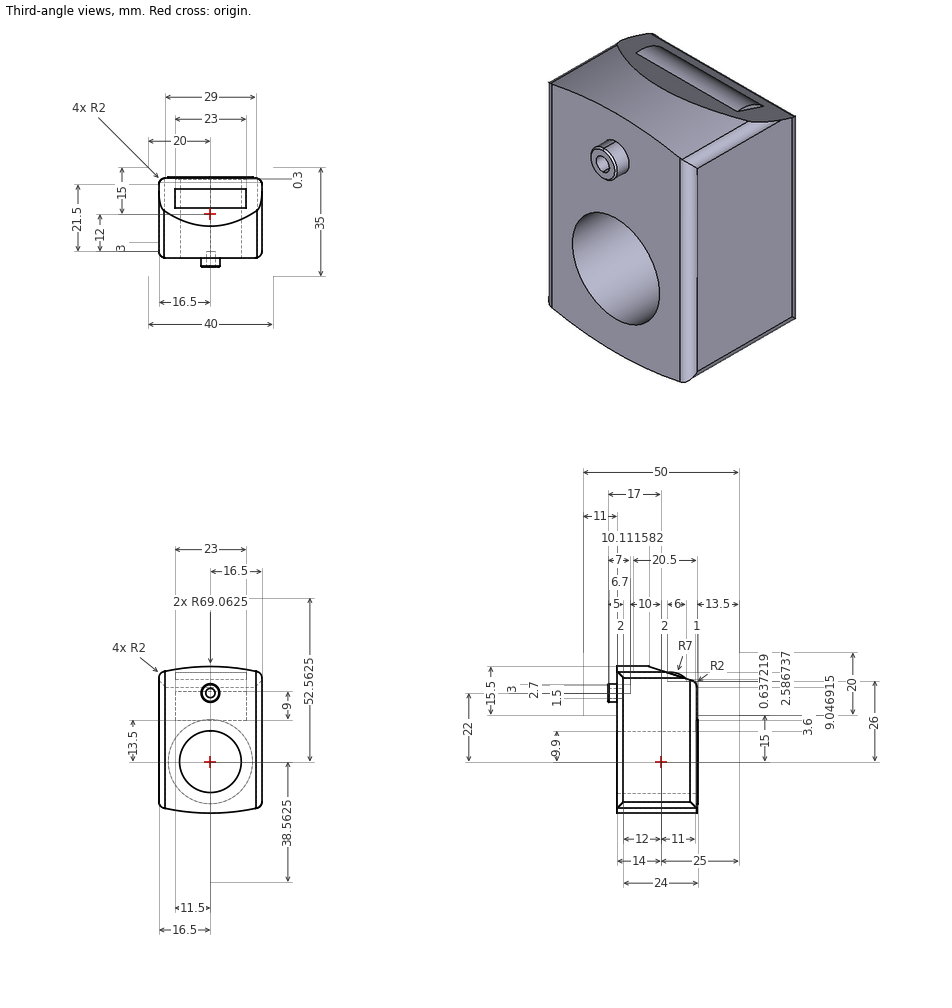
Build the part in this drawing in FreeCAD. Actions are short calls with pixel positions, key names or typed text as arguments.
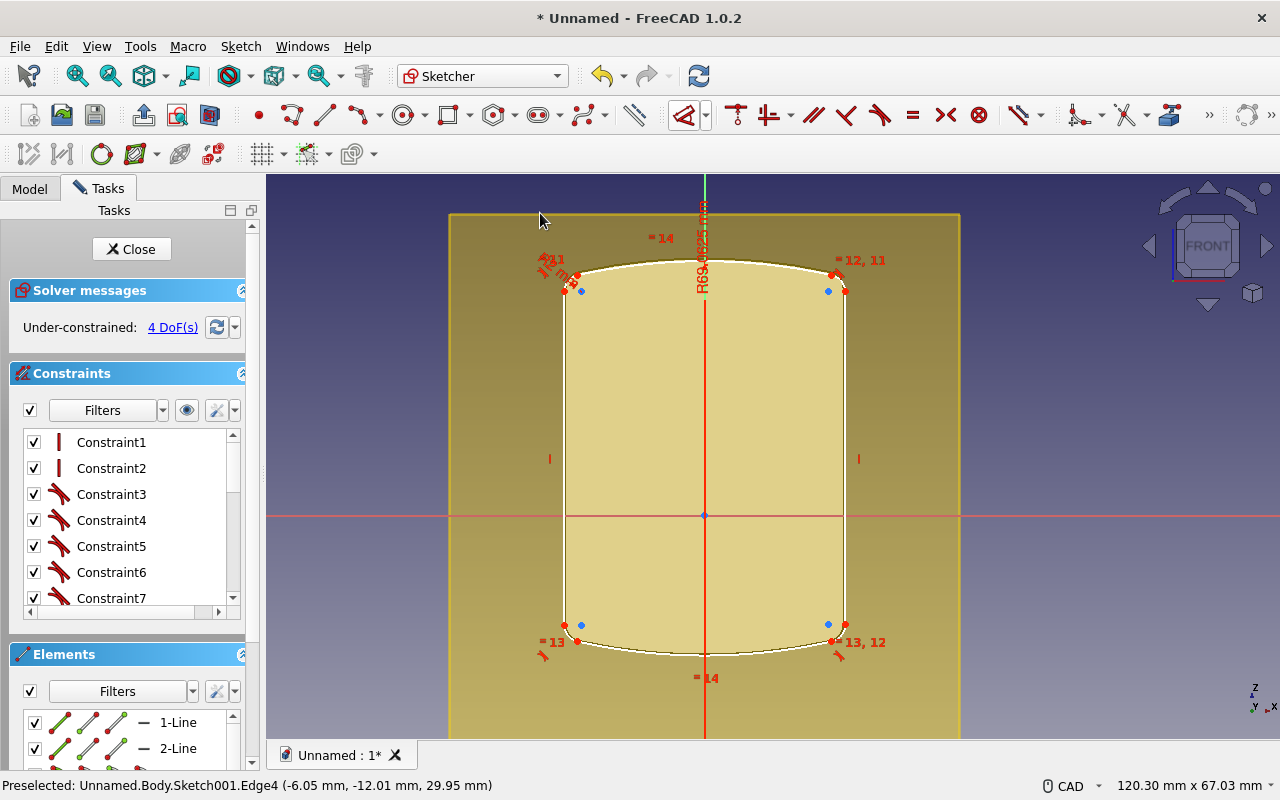
click(564, 625)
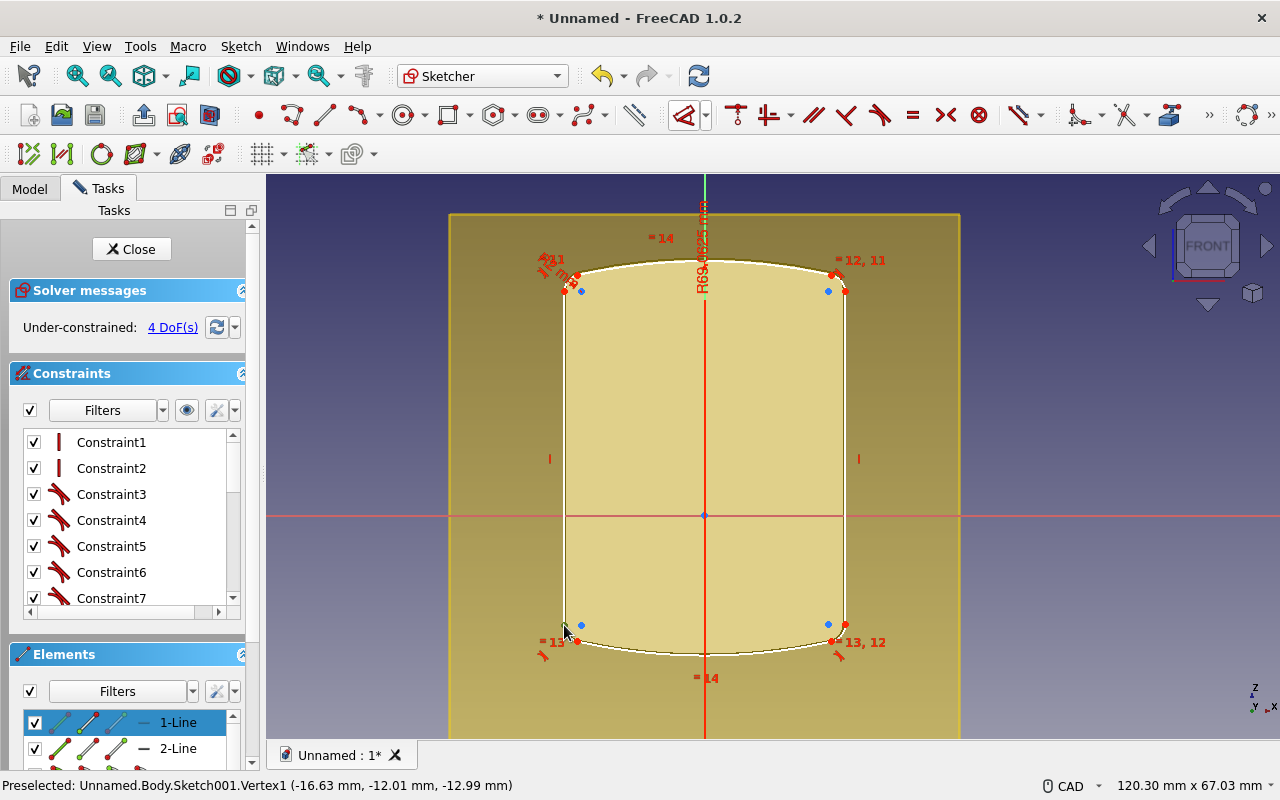
click(706, 116)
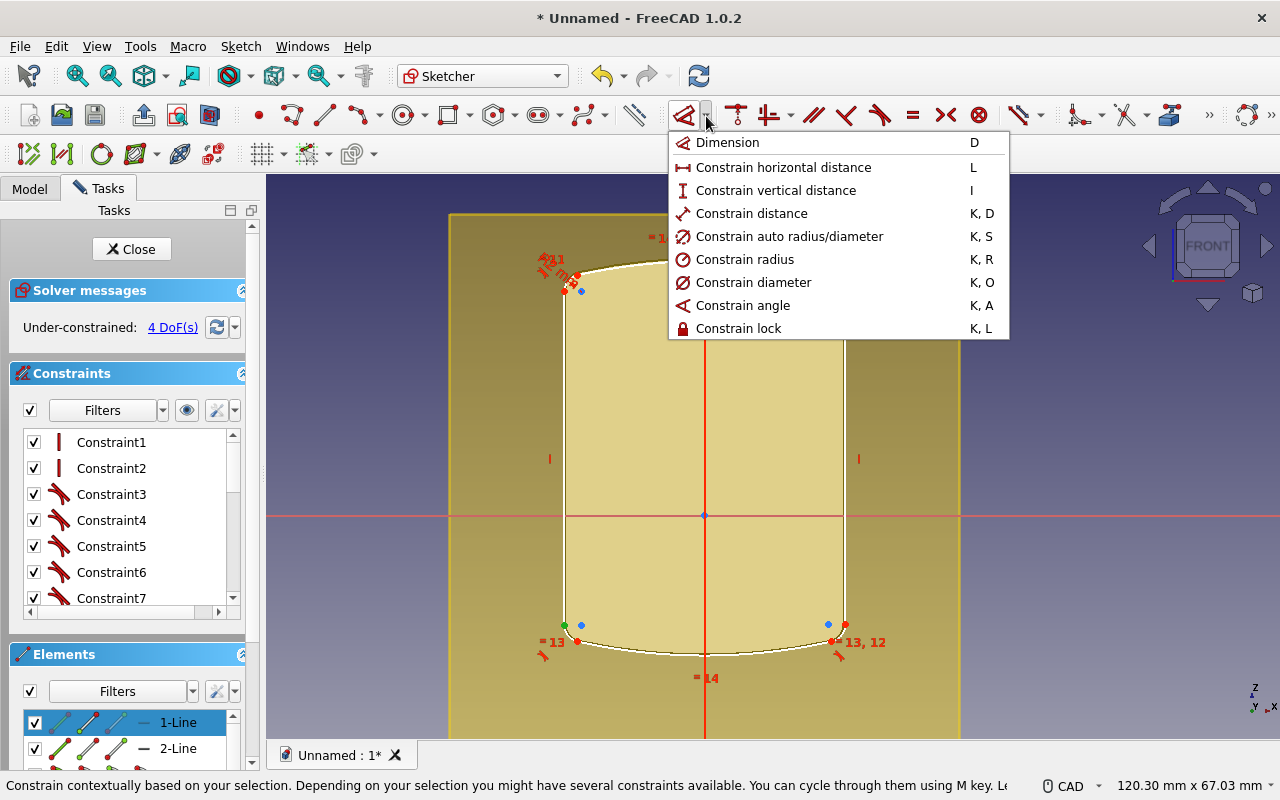
click(839, 168)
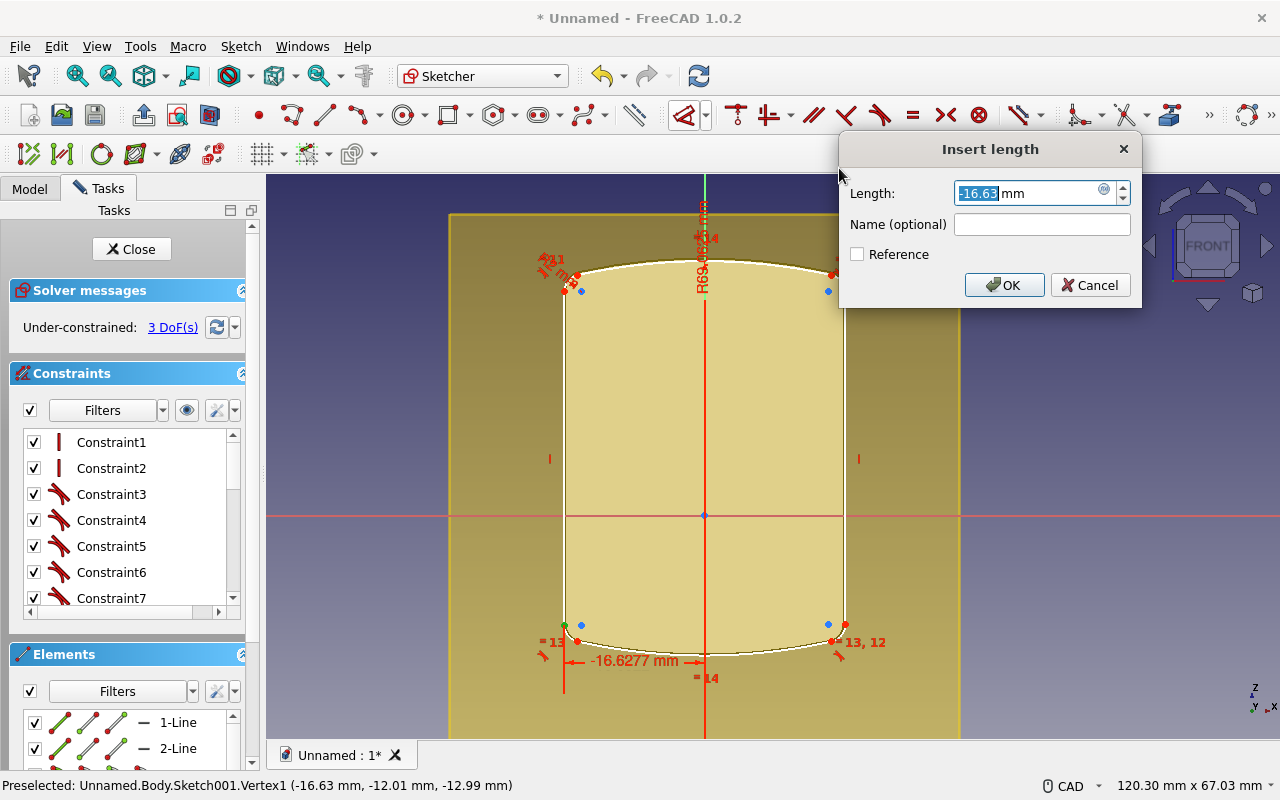
text(-16.5)
key(Return)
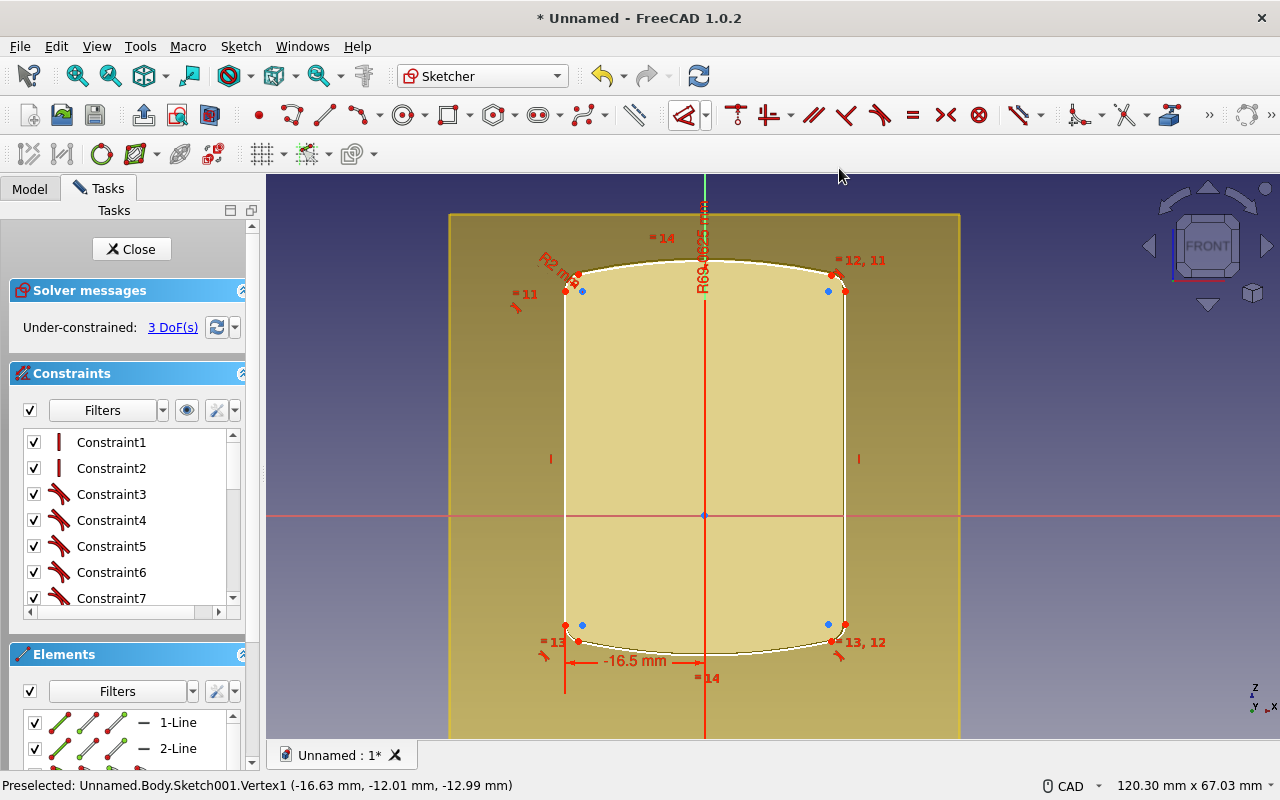
click(845, 292)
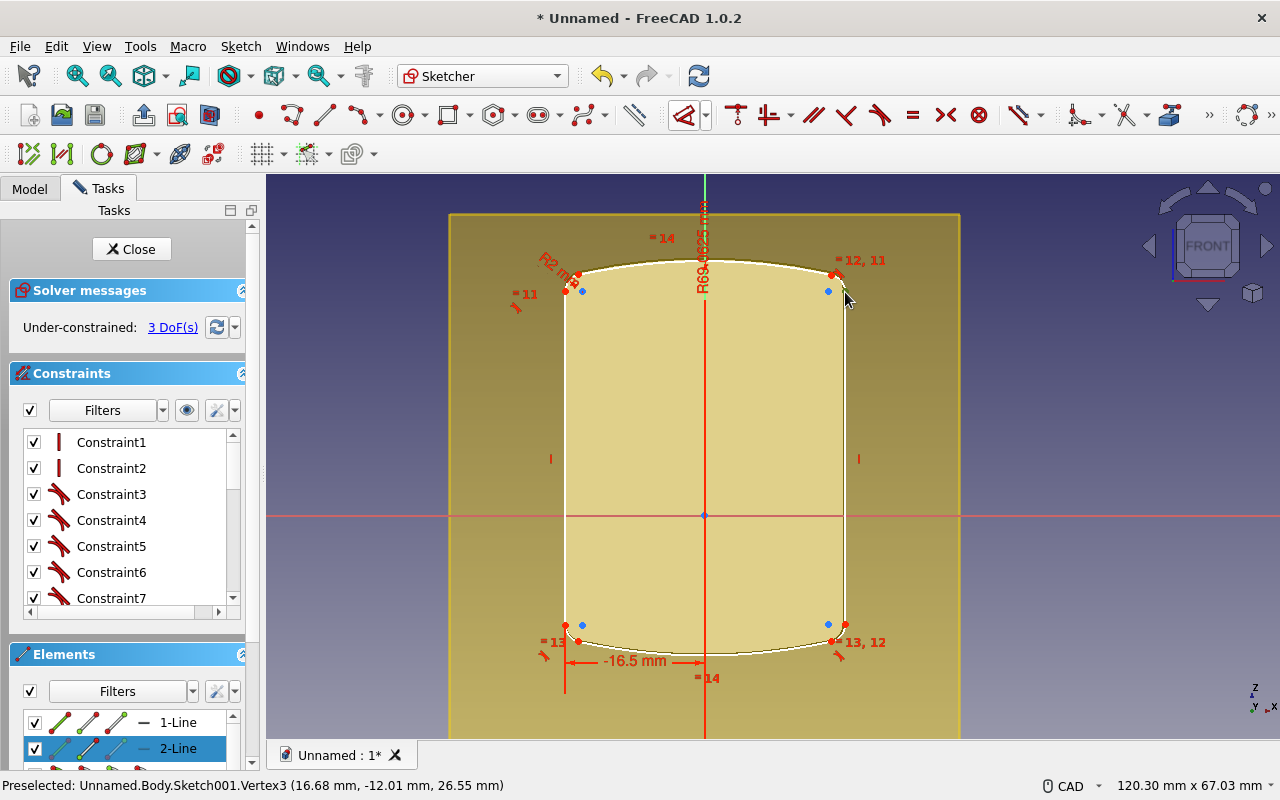
key(l)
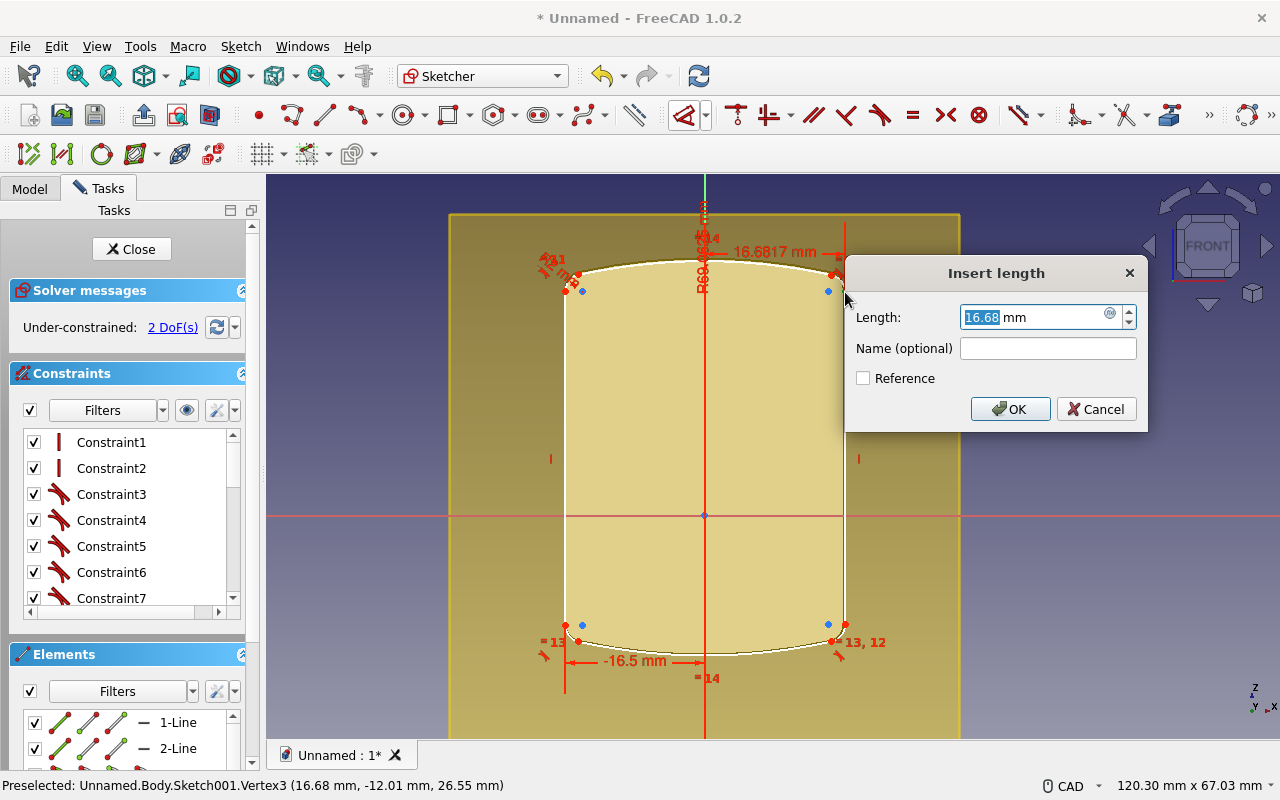
text(16.5)
key(Return)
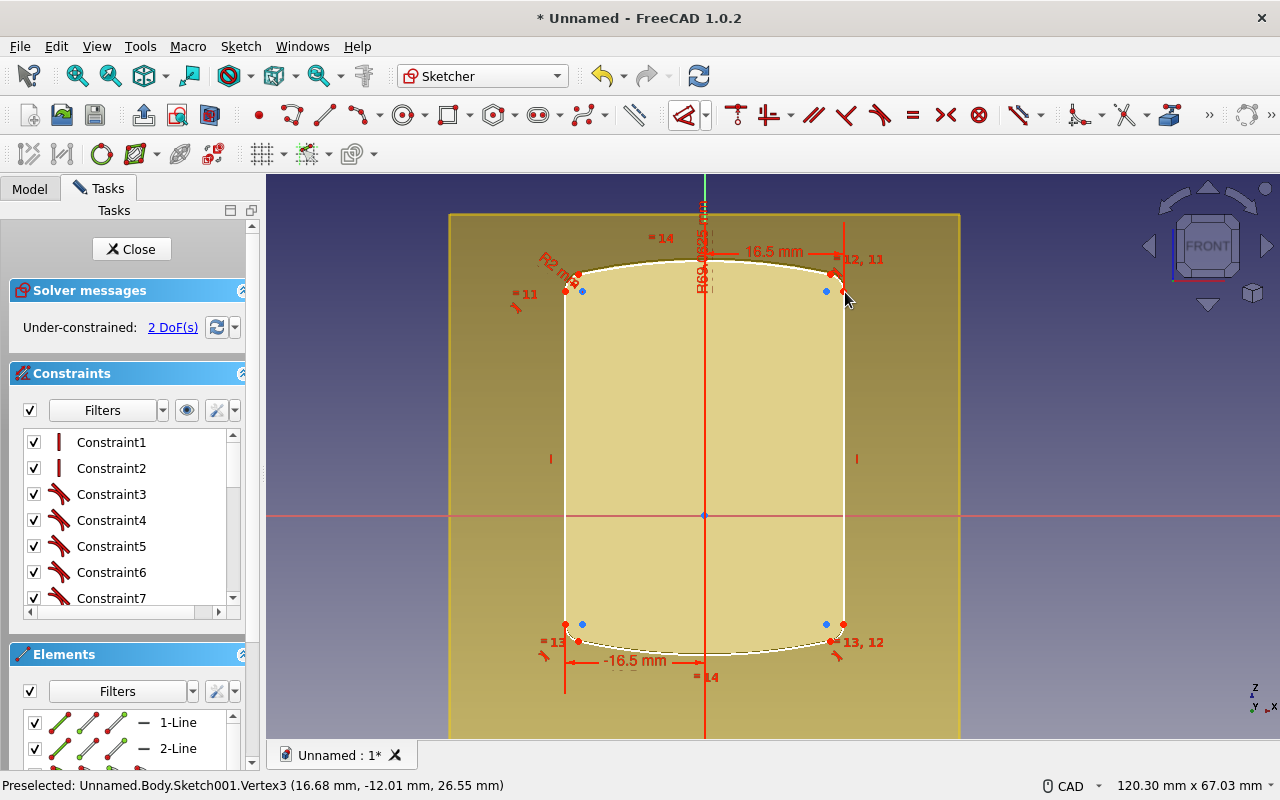
scroll(704, 265, down, 2)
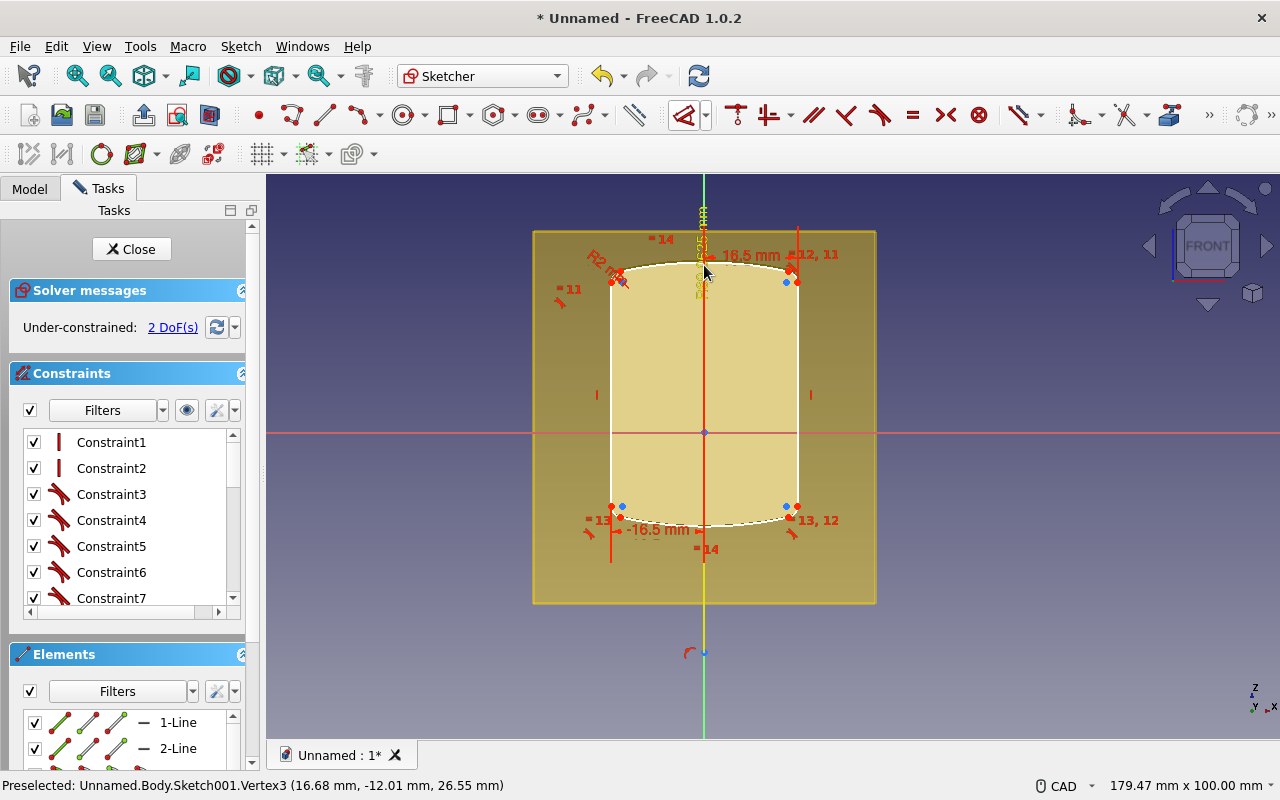
click(704, 653)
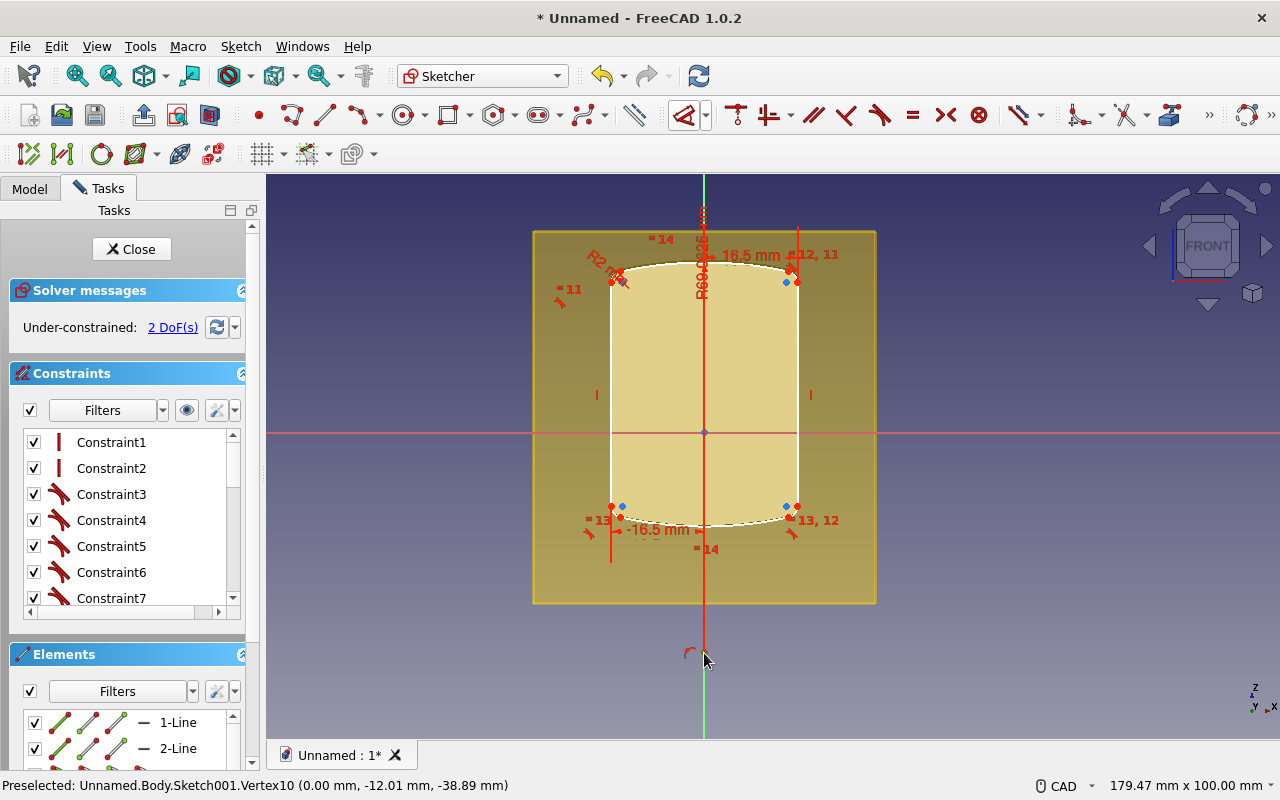
click(706, 116)